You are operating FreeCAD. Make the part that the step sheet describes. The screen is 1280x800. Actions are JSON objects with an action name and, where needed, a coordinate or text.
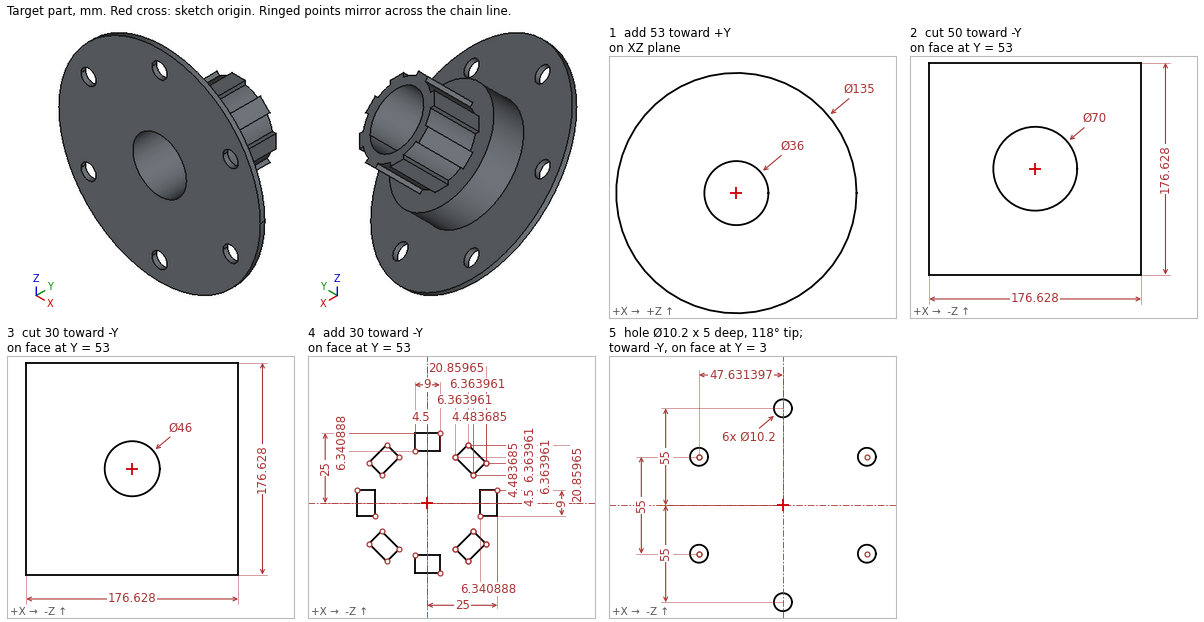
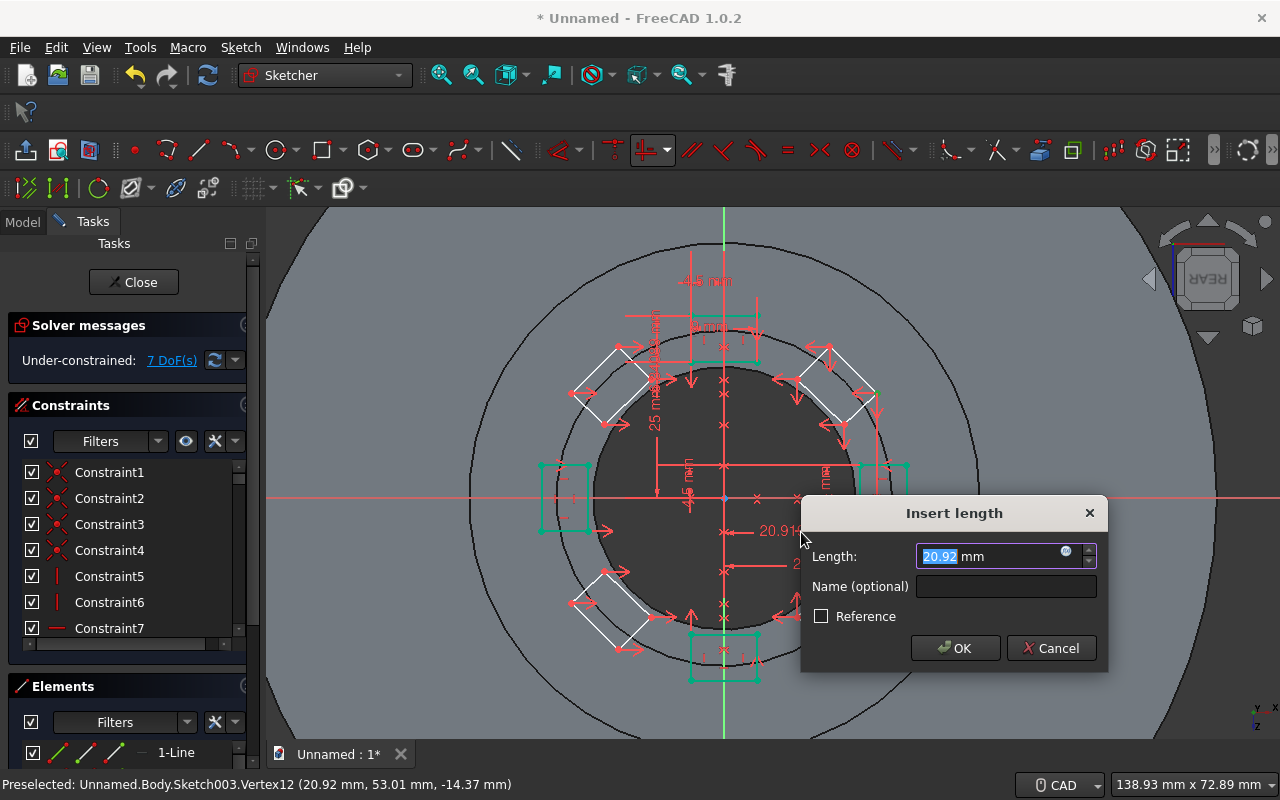
{"action": "type", "text": "20.85965"}
{"action": "key", "text": "Return"}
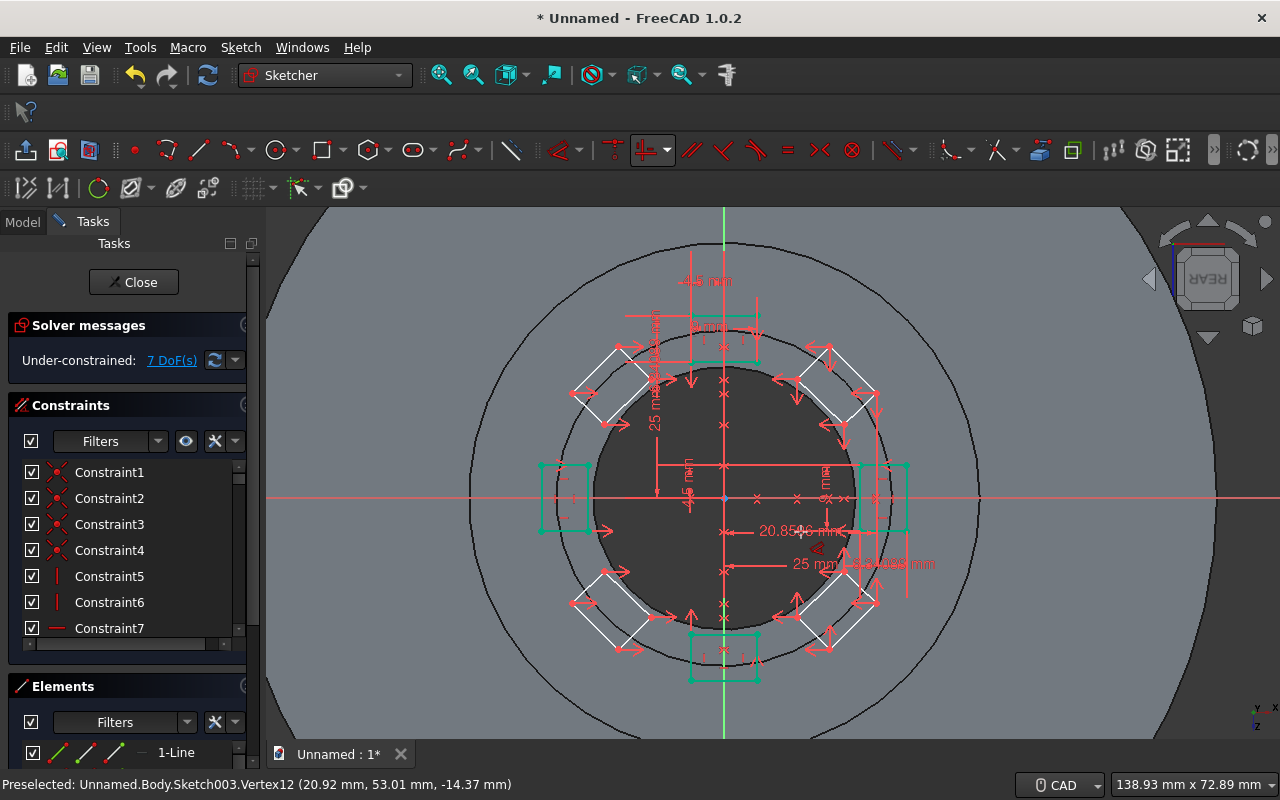
{"action": "left_click", "coordinate": [830, 347]}
{"action": "left_click", "coordinate": [690, 457]}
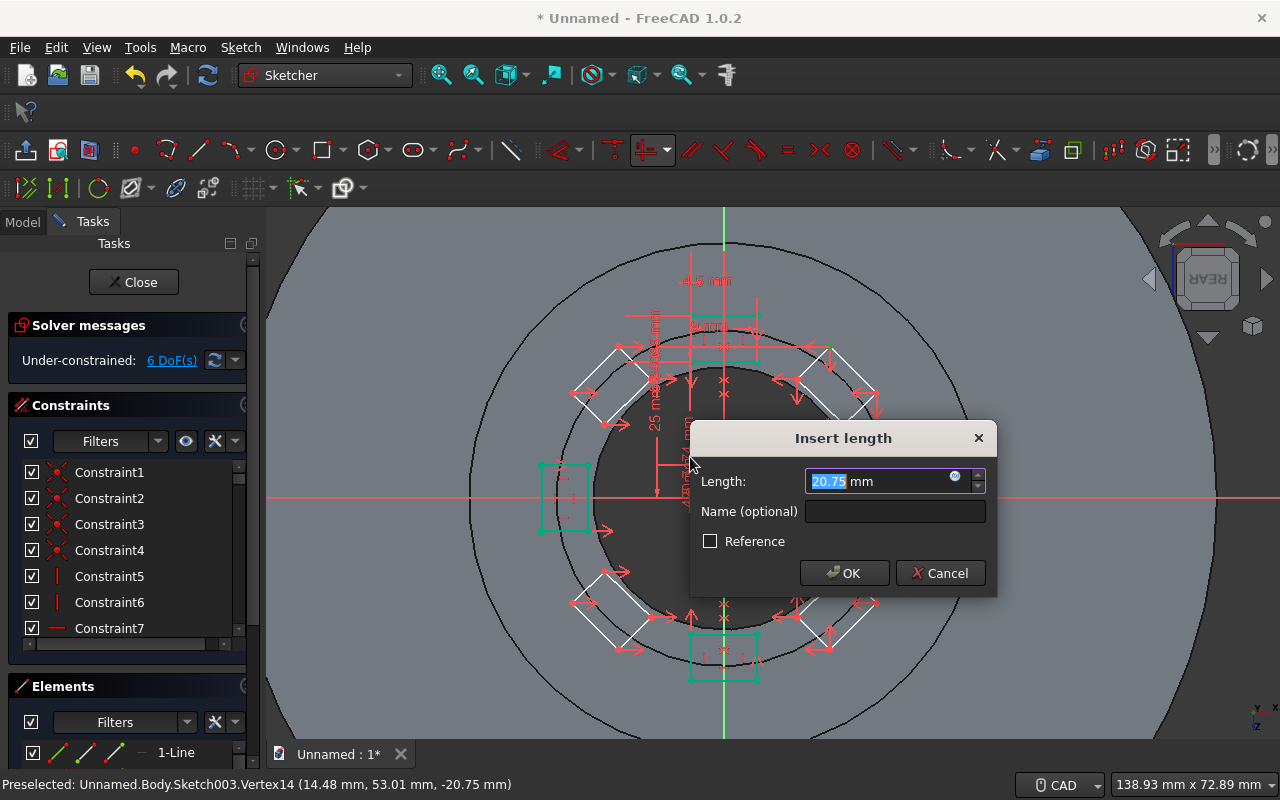
{"action": "type", "text": "20.85965"}
{"action": "key", "text": "Return"}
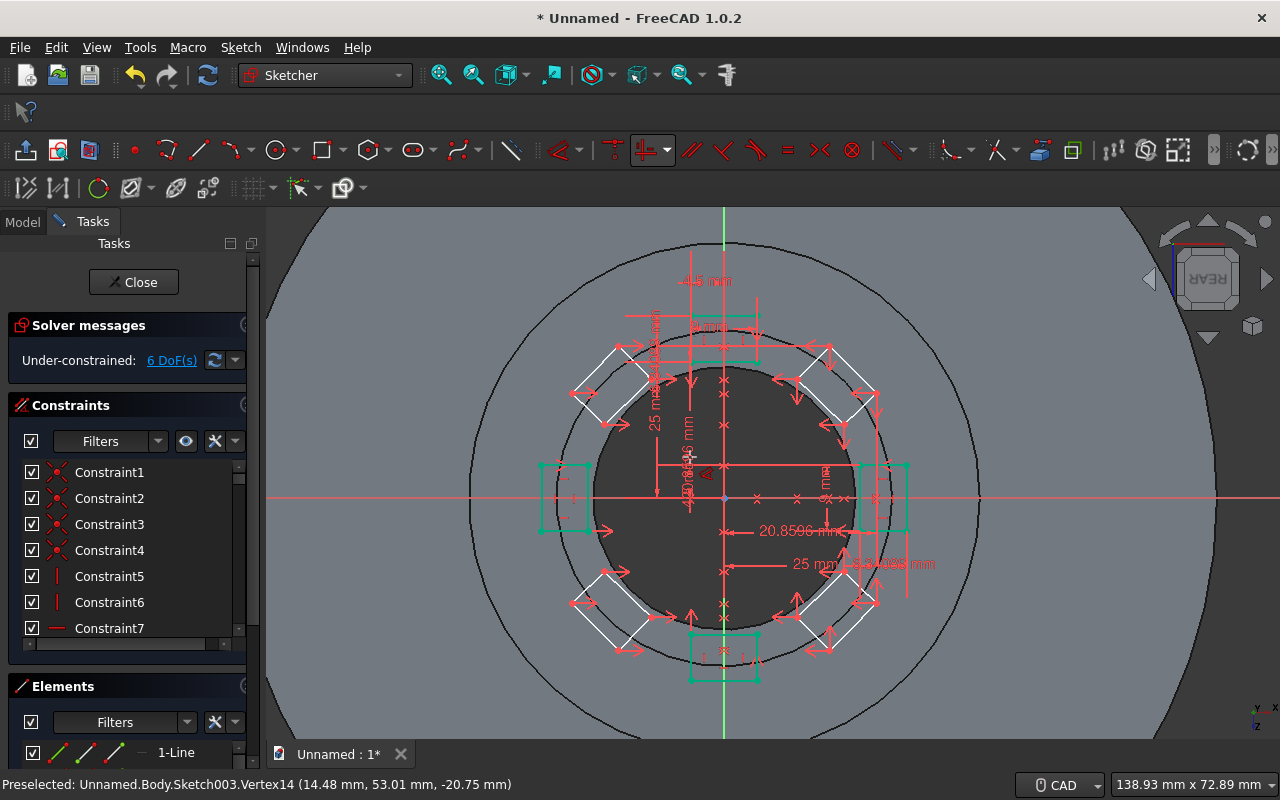
{"action": "left_click", "coordinate": [811, 393]}
{"action": "left_click", "coordinate": [810, 345]}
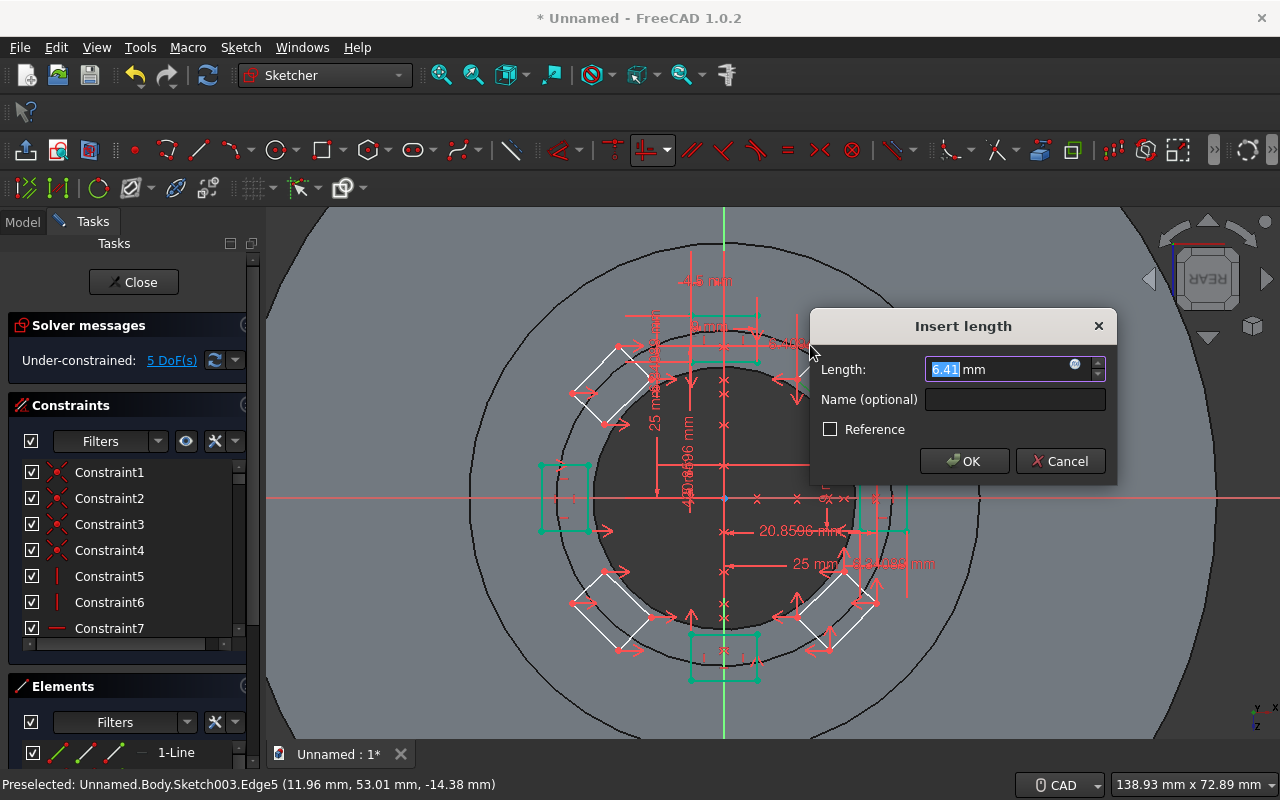
{"action": "type", "text": "6.363961"}
{"action": "key", "text": "Return"}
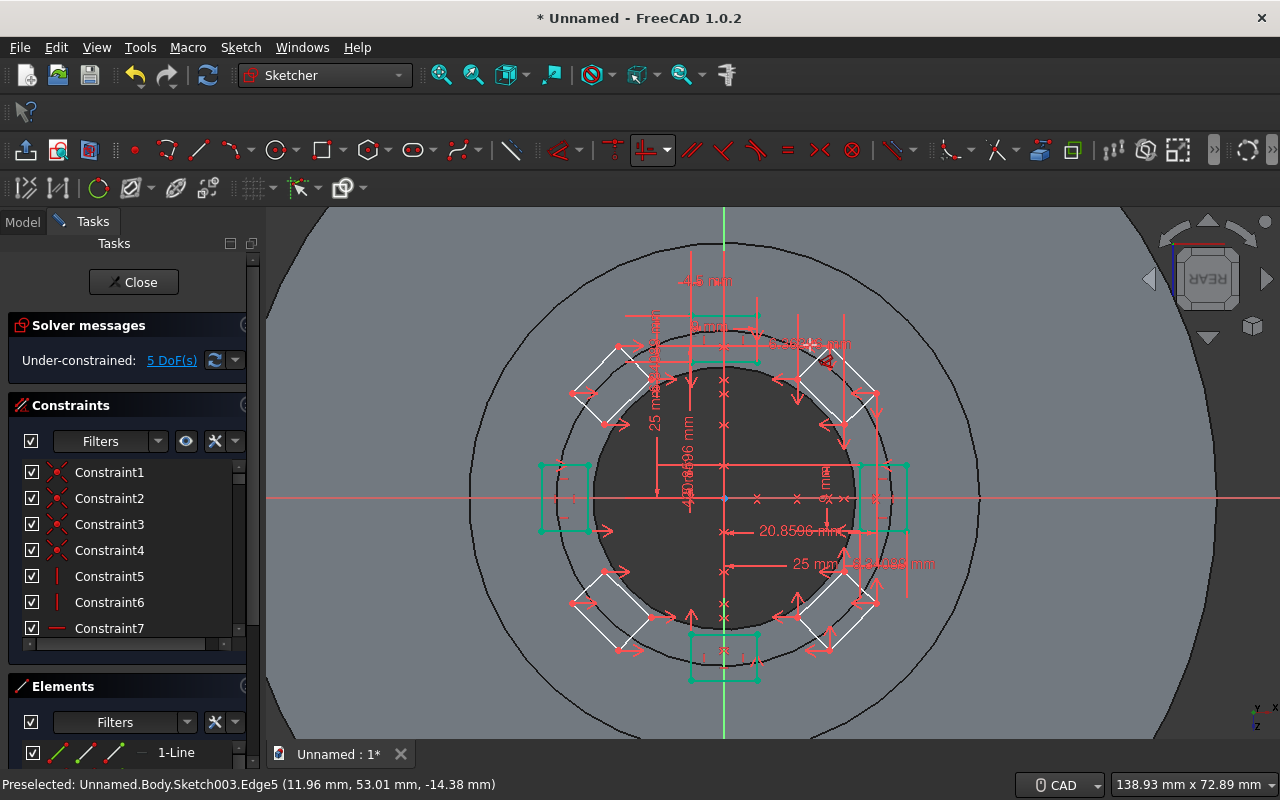
{"action": "left_click", "coordinate": [811, 393]}
{"action": "left_click", "coordinate": [878, 412]}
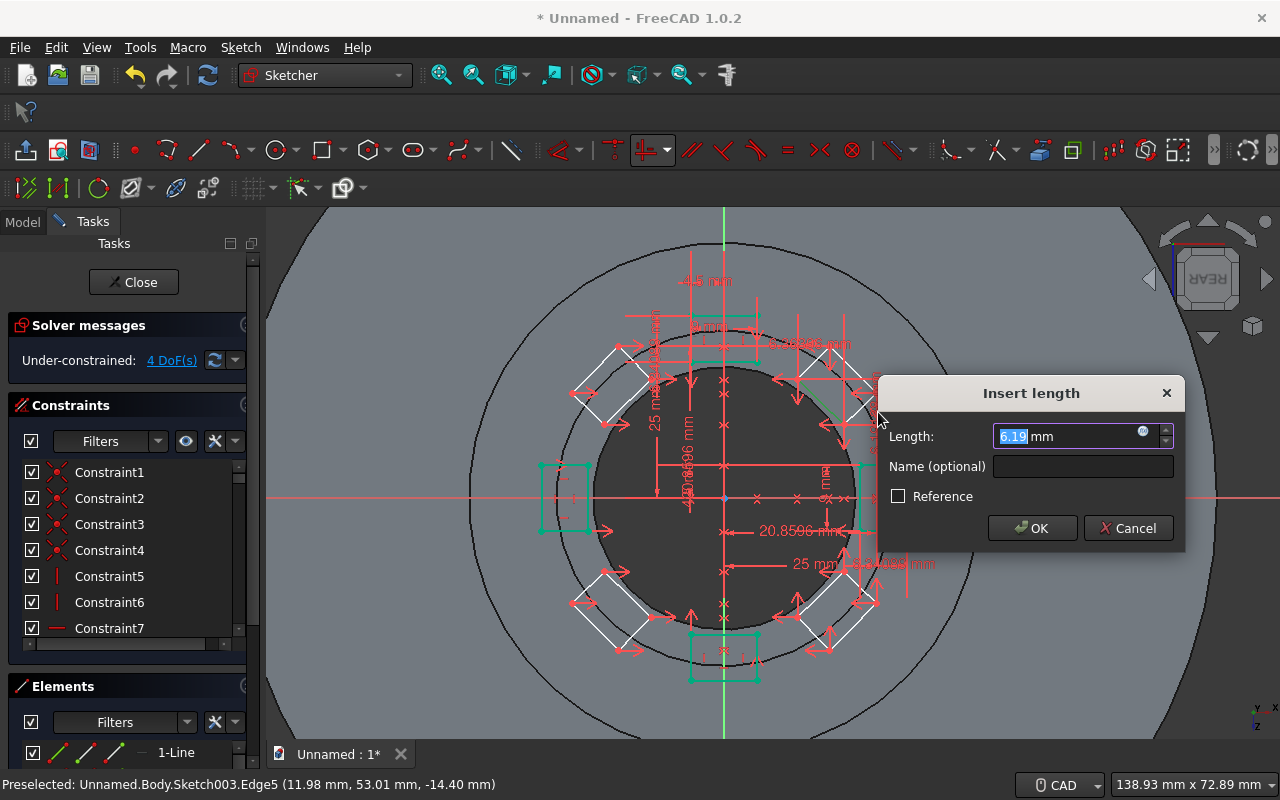
{"action": "type", "text": "6.363961"}
{"action": "key", "text": "Return"}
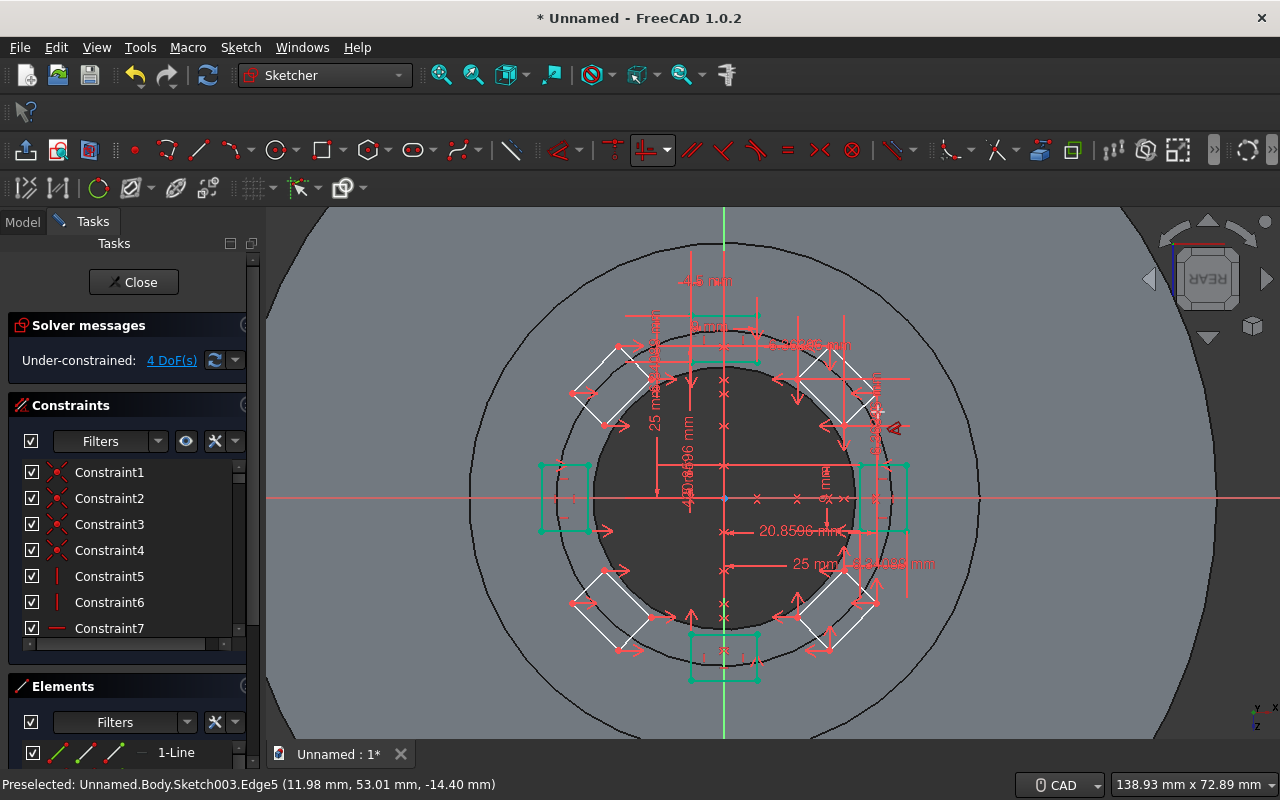
{"action": "left_click", "coordinate": [854, 416]}
{"action": "left_click", "coordinate": [860, 311]}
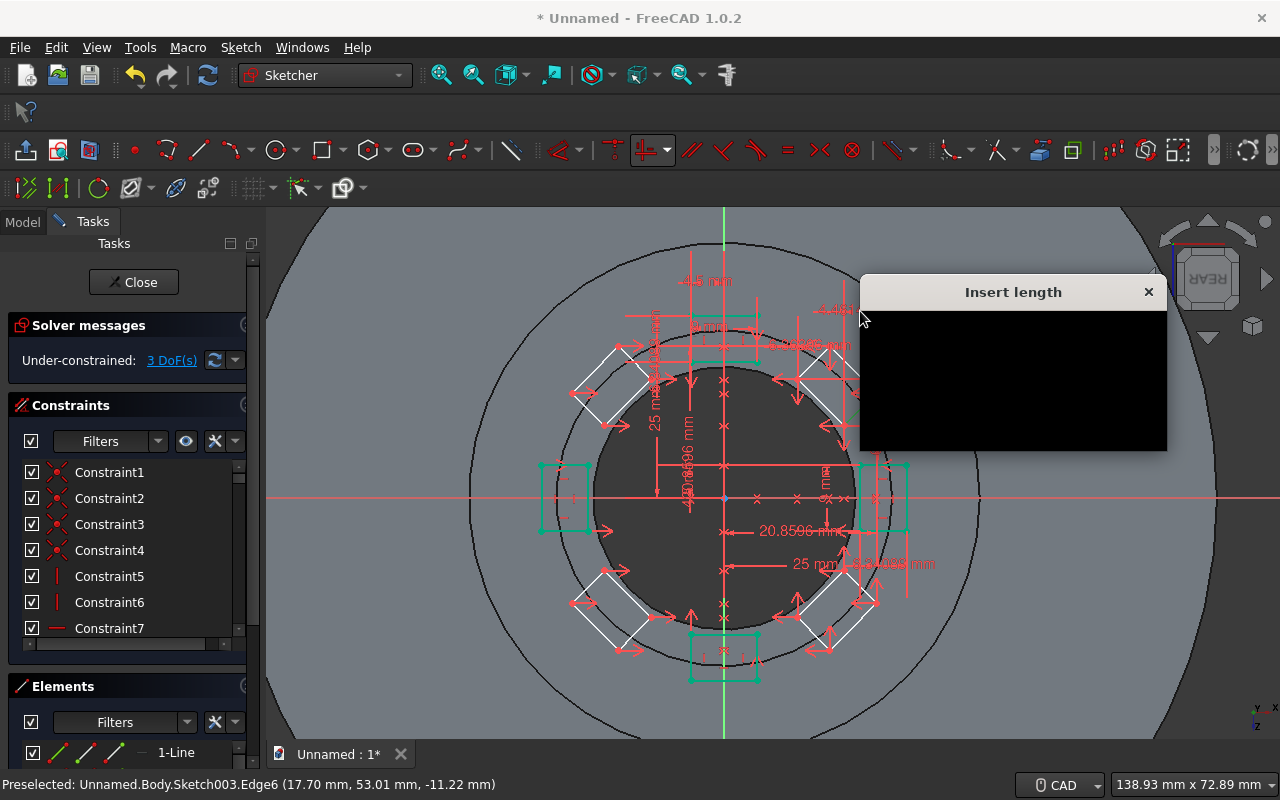
{"action": "type", "text": "4.483685"}
{"action": "key", "text": "Return"}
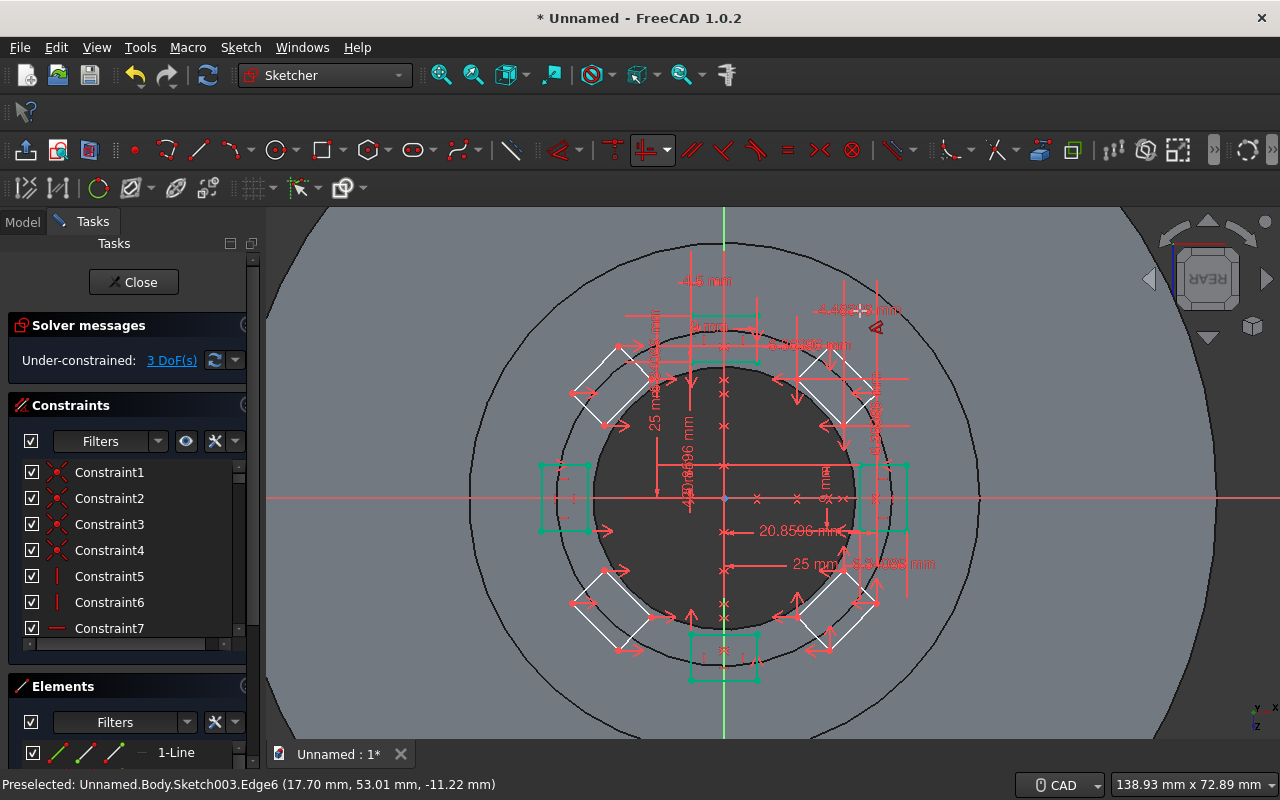
{"action": "left_click", "coordinate": [854, 416]}
{"action": "left_click", "coordinate": [786, 410]}